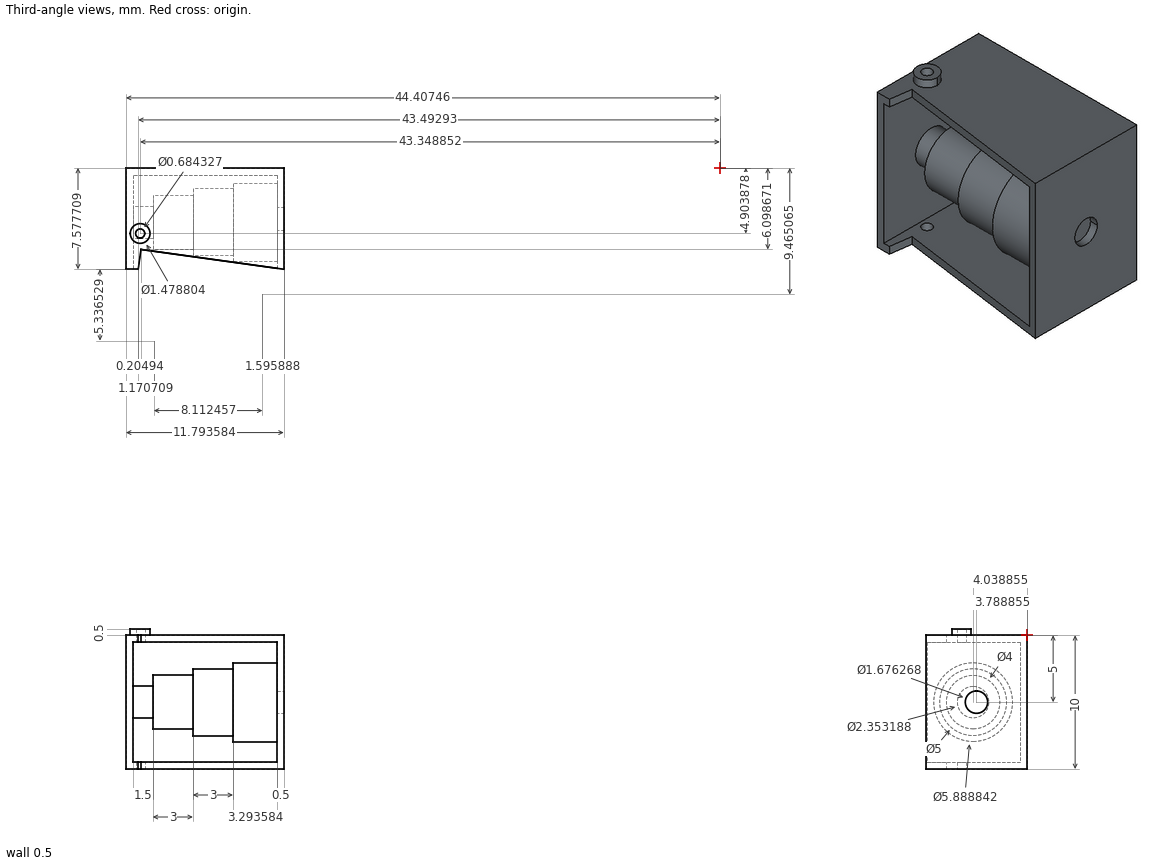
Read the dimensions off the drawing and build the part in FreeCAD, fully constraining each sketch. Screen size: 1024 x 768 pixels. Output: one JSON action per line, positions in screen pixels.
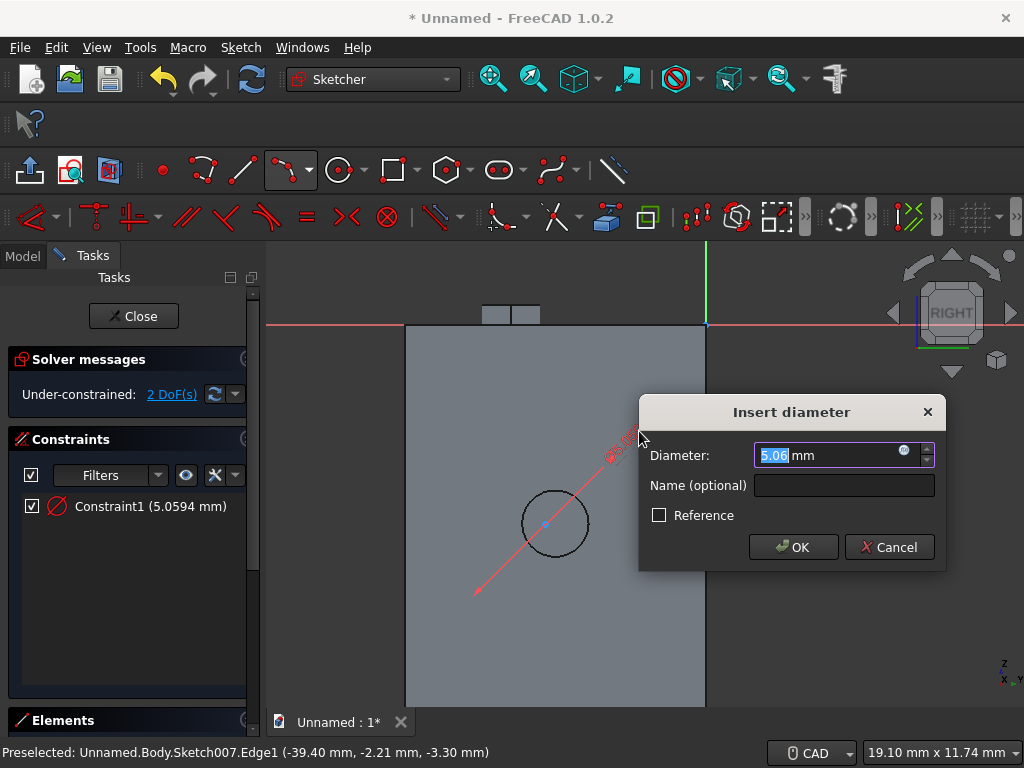
{"action": "type", "text": "5"}
{"action": "key", "text": "Return"}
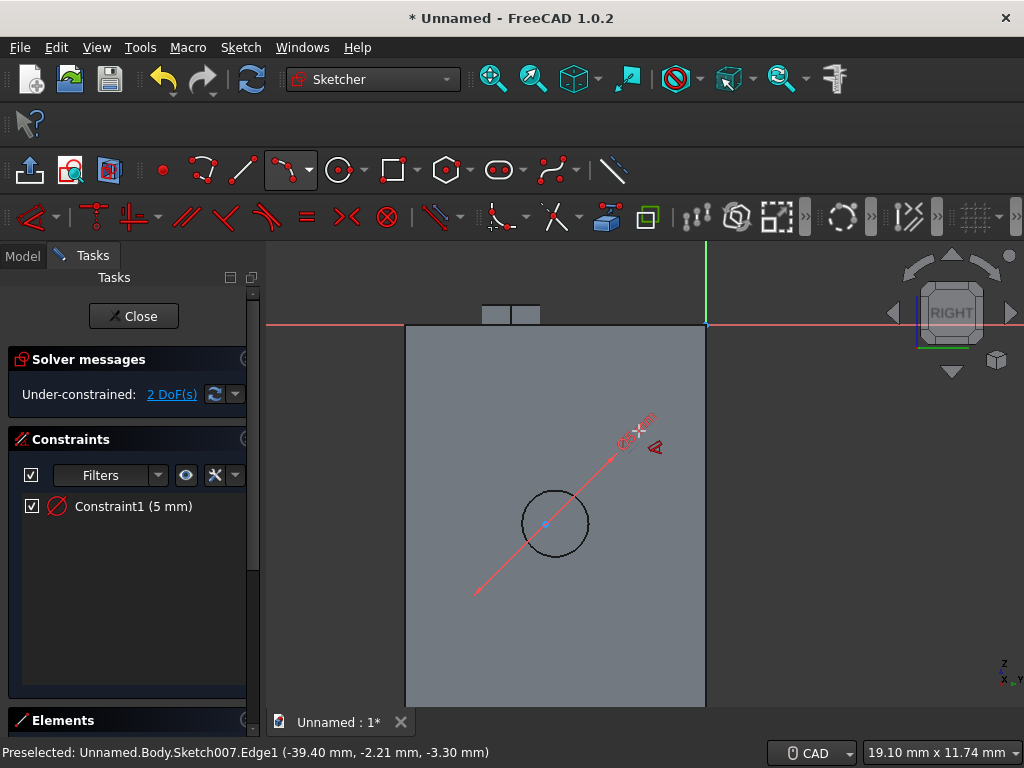
{"action": "left_click", "coordinate": [545, 525]}
{"action": "left_click", "coordinate": [740, 425]}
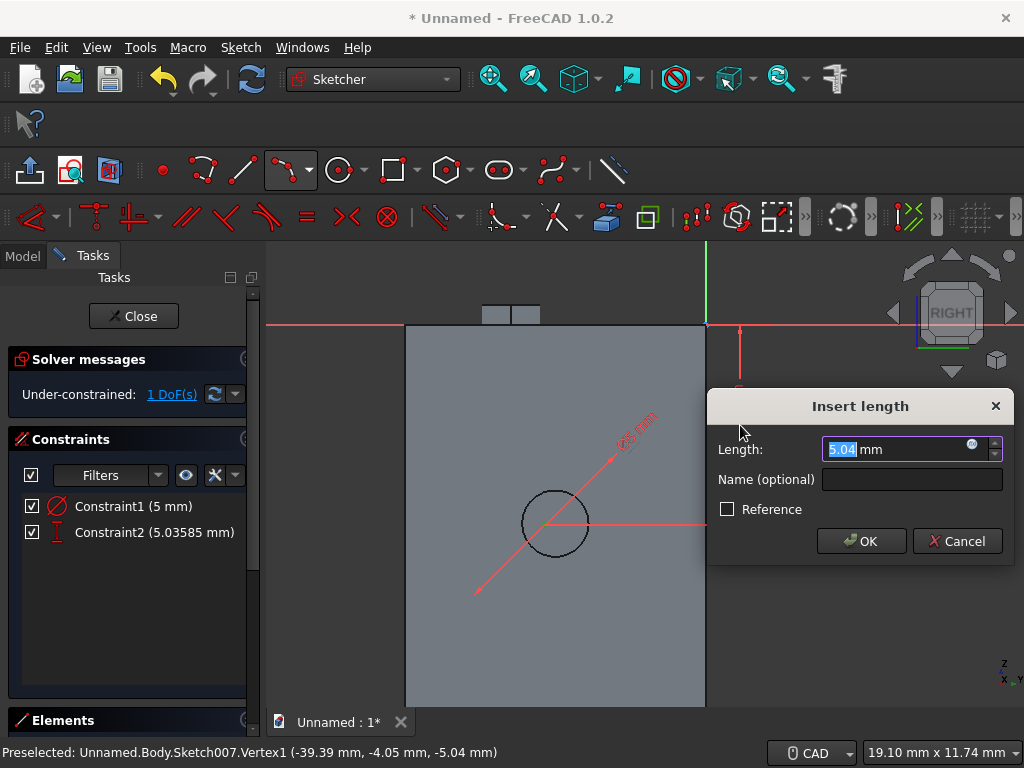
{"action": "type", "text": "5"}
{"action": "key", "text": "Return"}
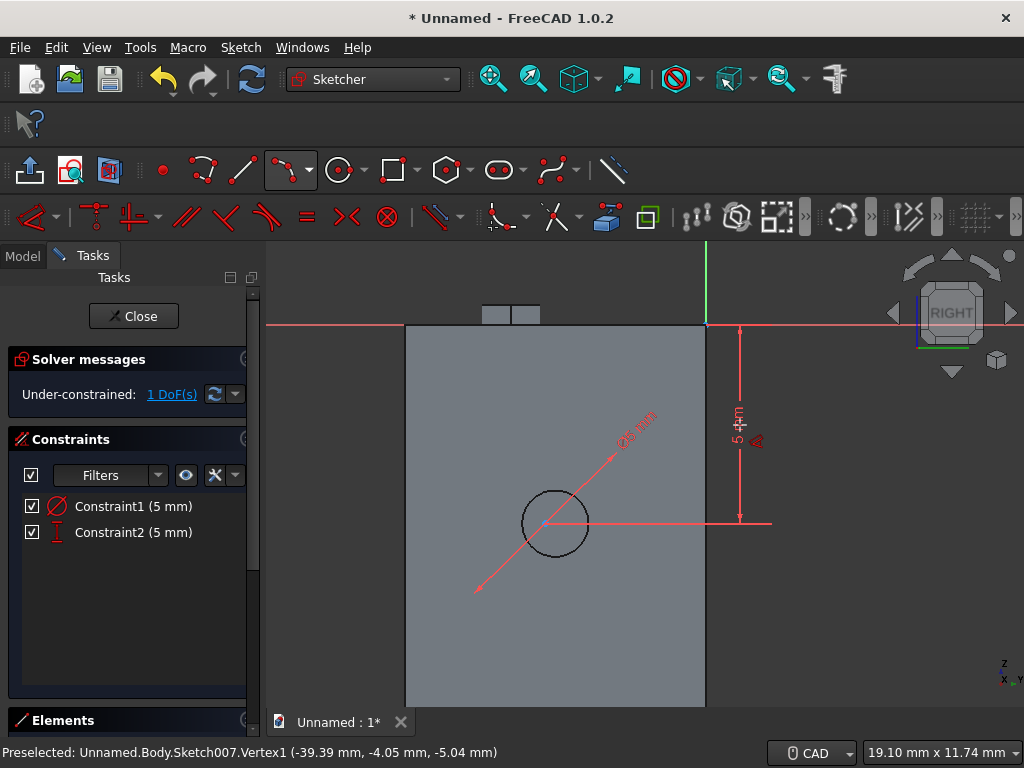
{"action": "left_click", "coordinate": [545, 524]}
{"action": "left_click", "coordinate": [625, 291]}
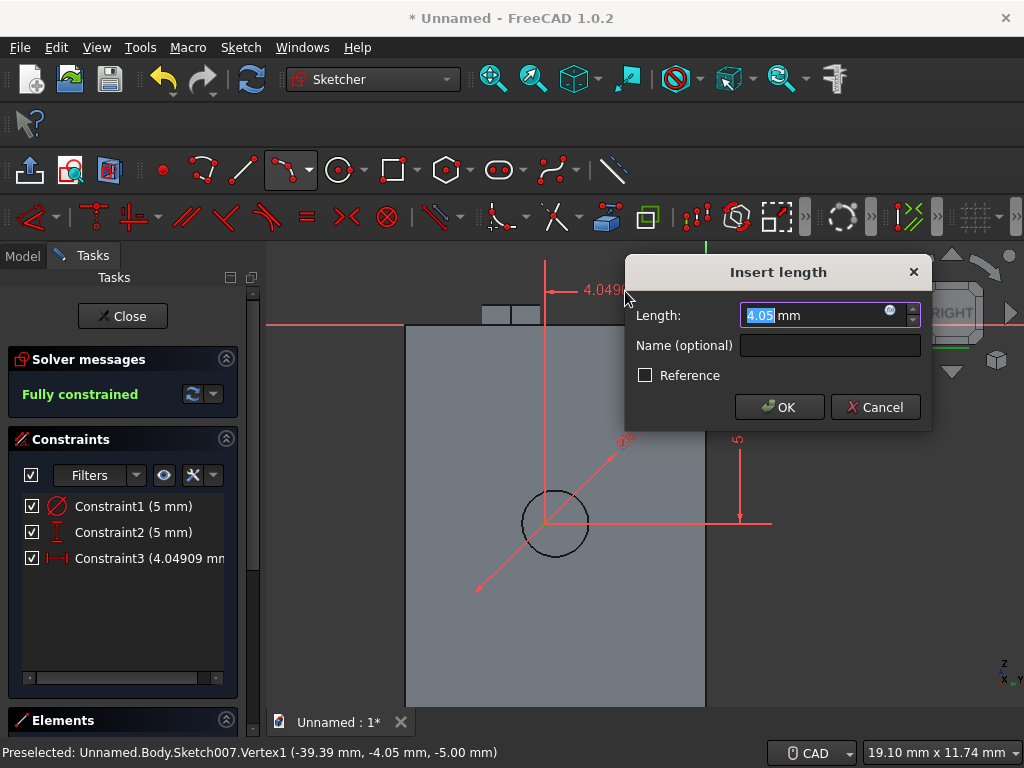
{"action": "type", "text": "4.038855"}
{"action": "key", "text": "Return"}
{"action": "key", "text": "Escape"}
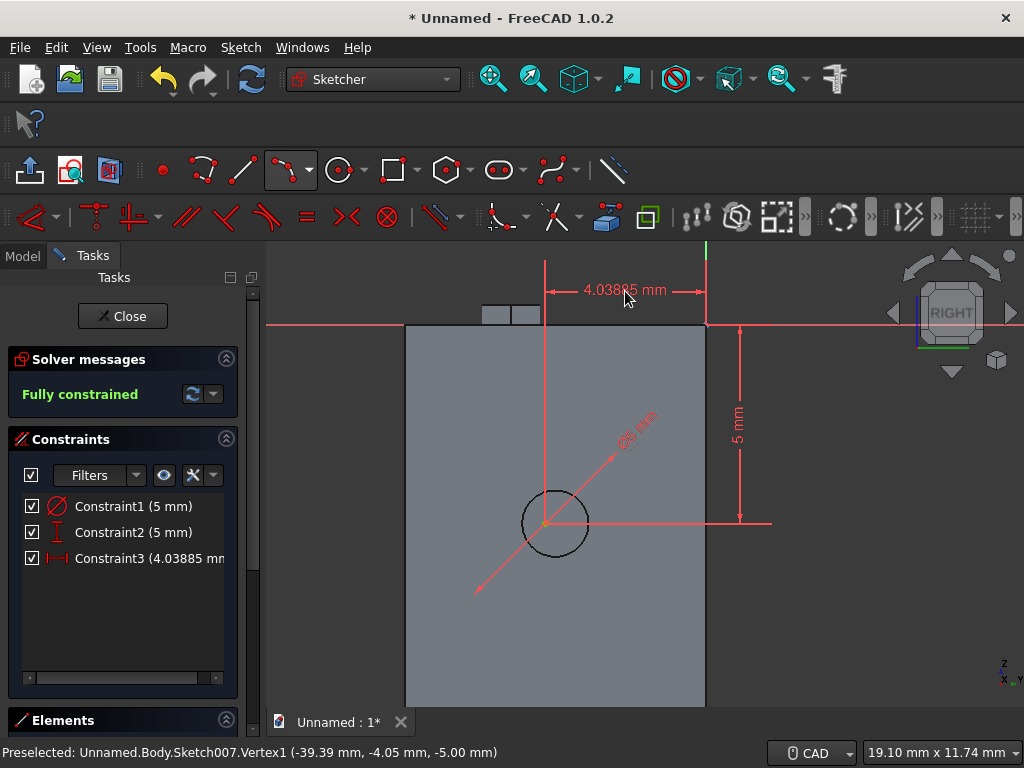
{"action": "left_click", "coordinate": [123, 316]}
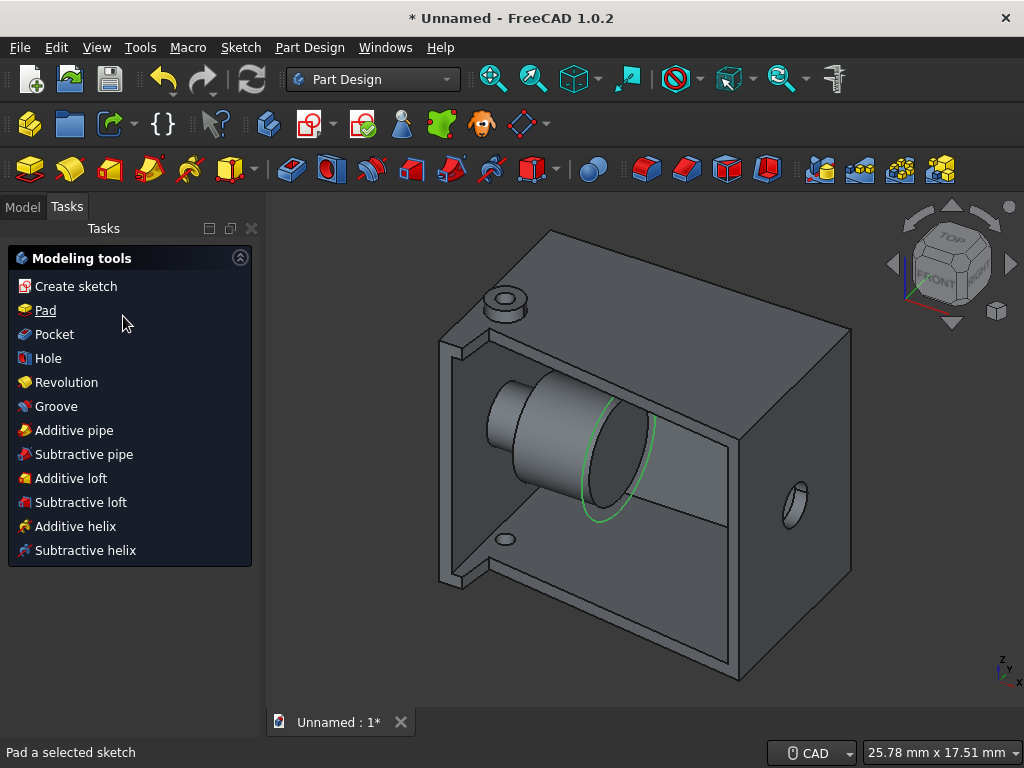
{"action": "left_click", "coordinate": [30, 170]}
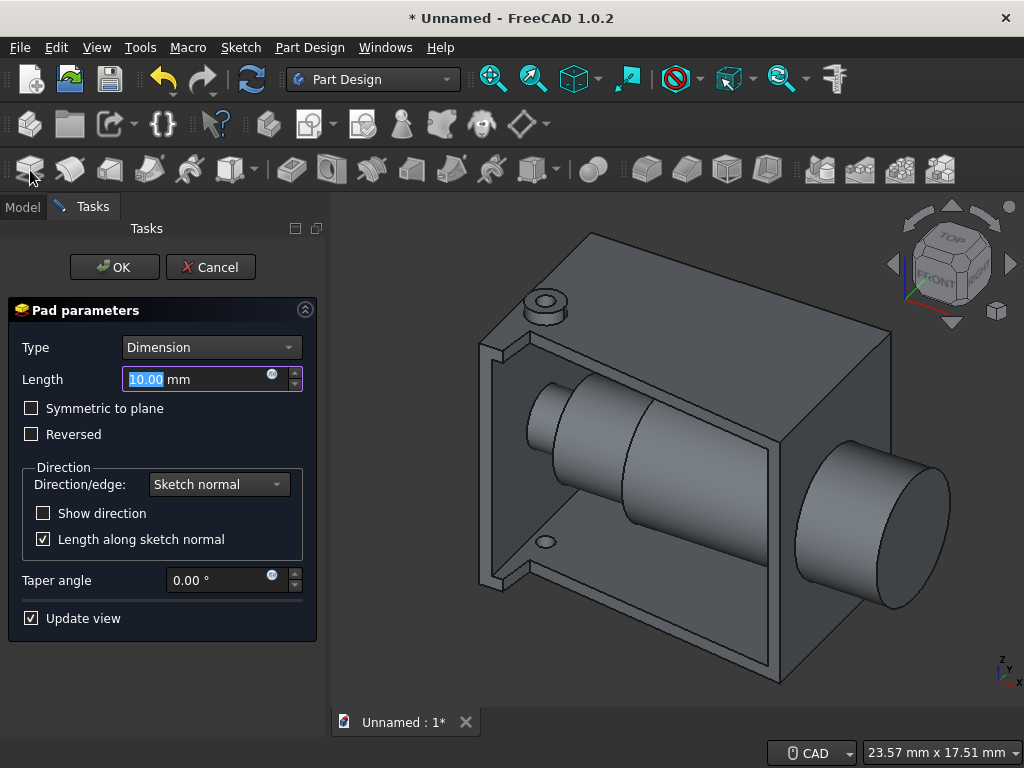
{"action": "type", "text": "3"}
{"action": "key", "text": "Tab"}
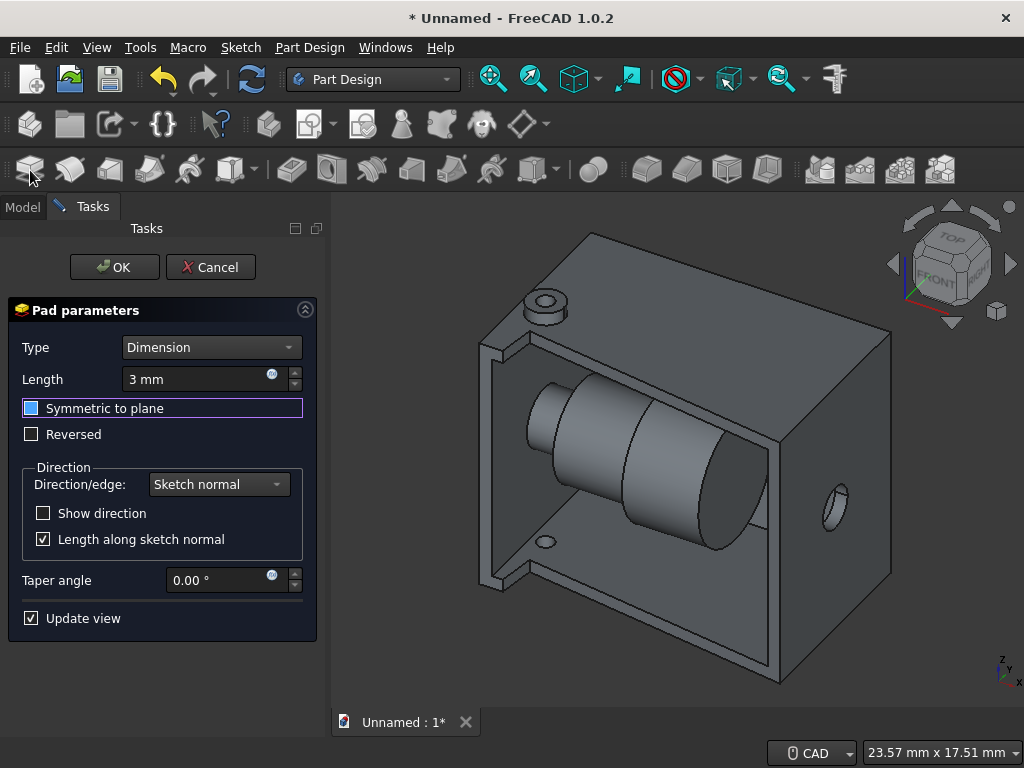
{"action": "left_click", "coordinate": [115, 267]}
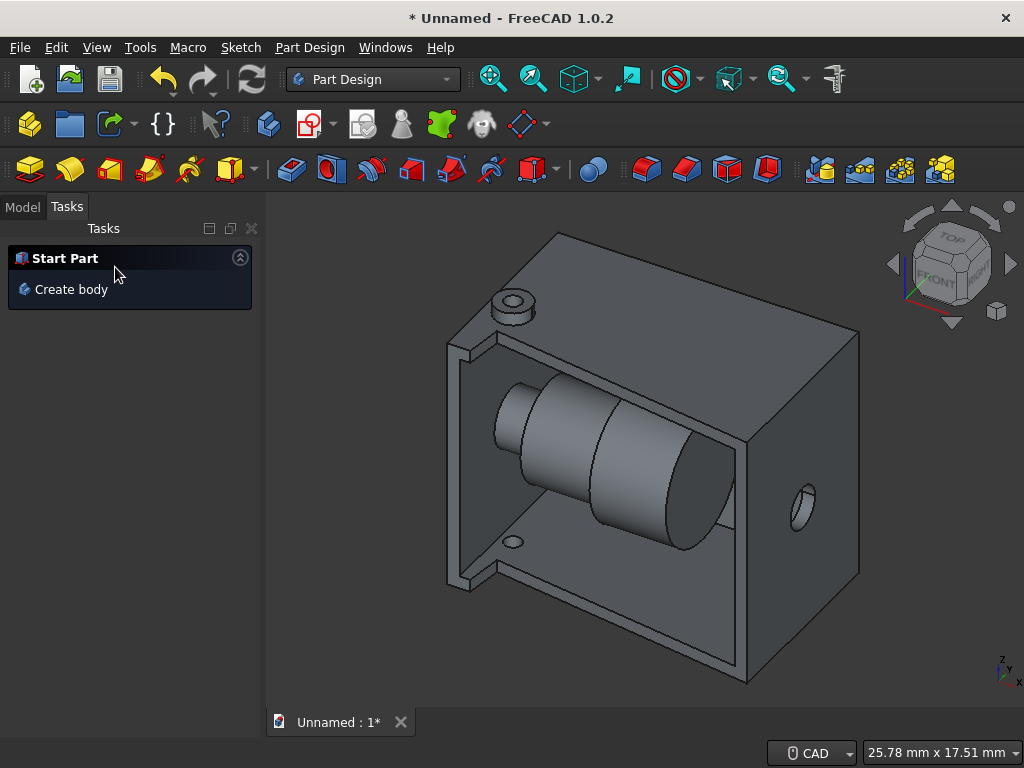
{"action": "left_click", "coordinate": [703, 478]}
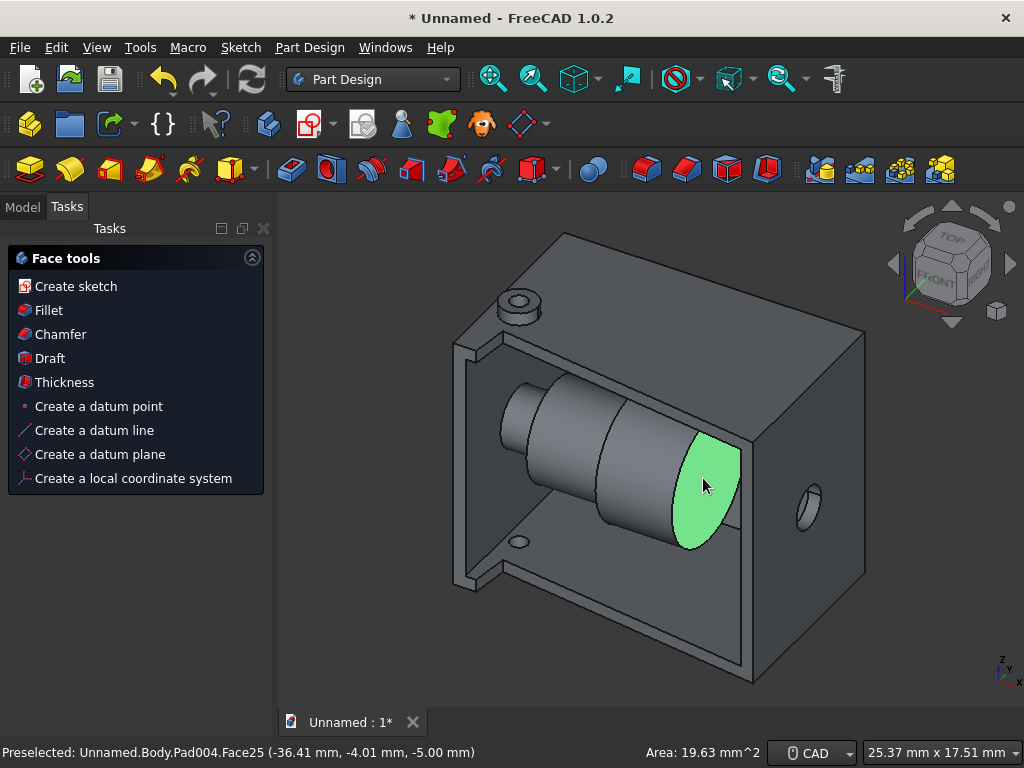
{"action": "left_click", "coordinate": [310, 124]}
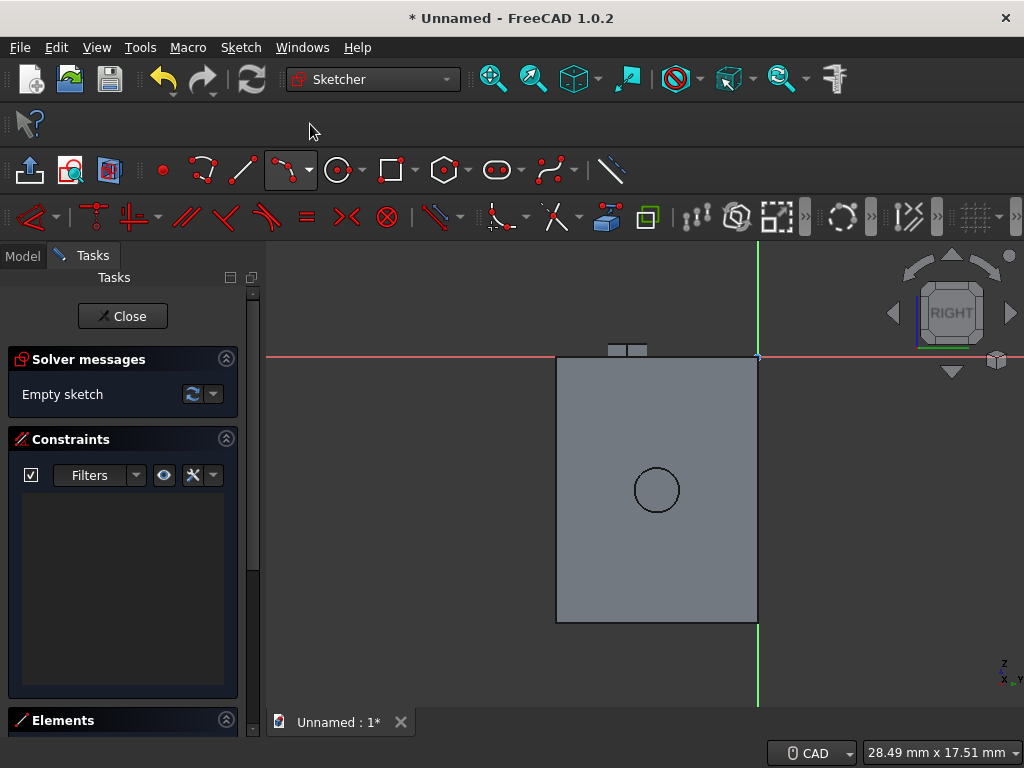
{"action": "left_click", "coordinate": [110, 170]}